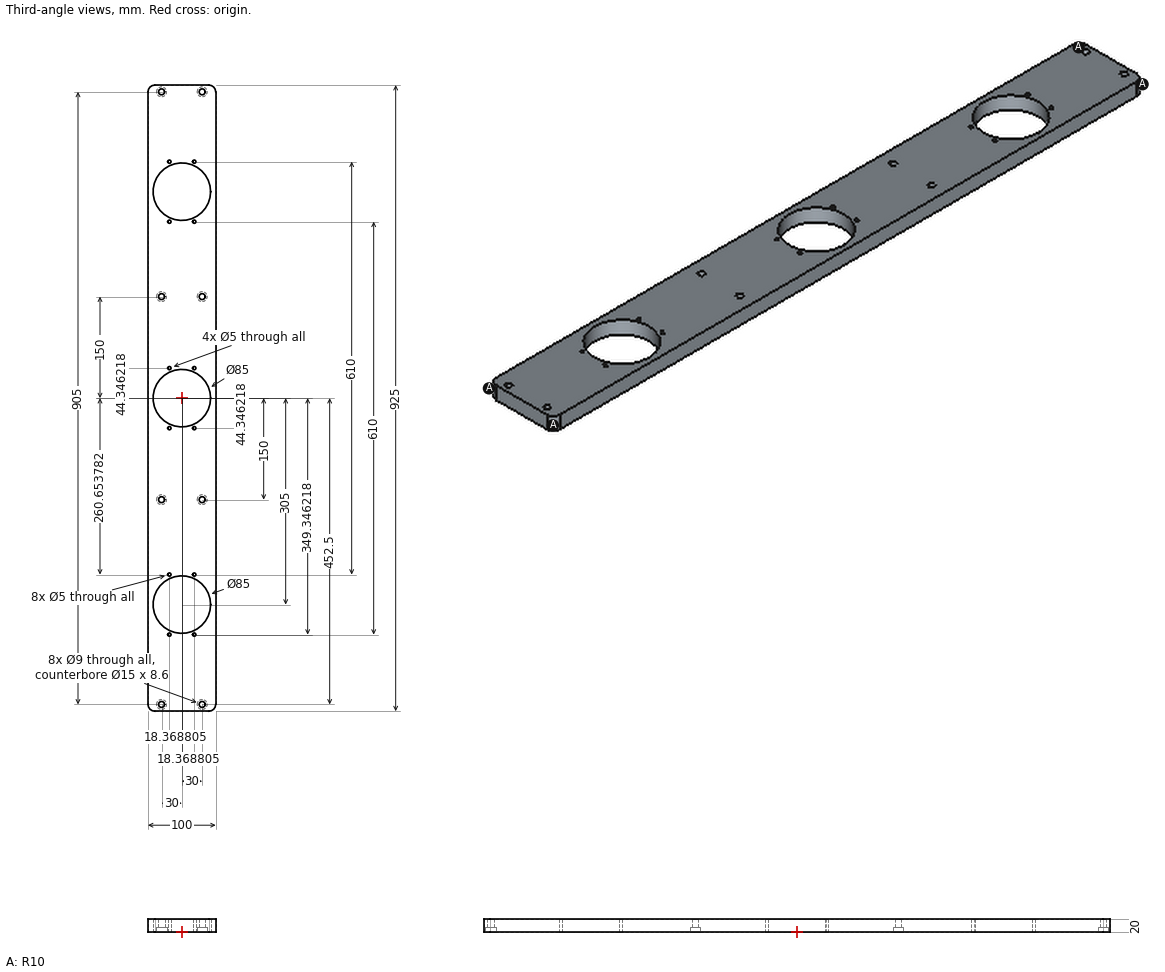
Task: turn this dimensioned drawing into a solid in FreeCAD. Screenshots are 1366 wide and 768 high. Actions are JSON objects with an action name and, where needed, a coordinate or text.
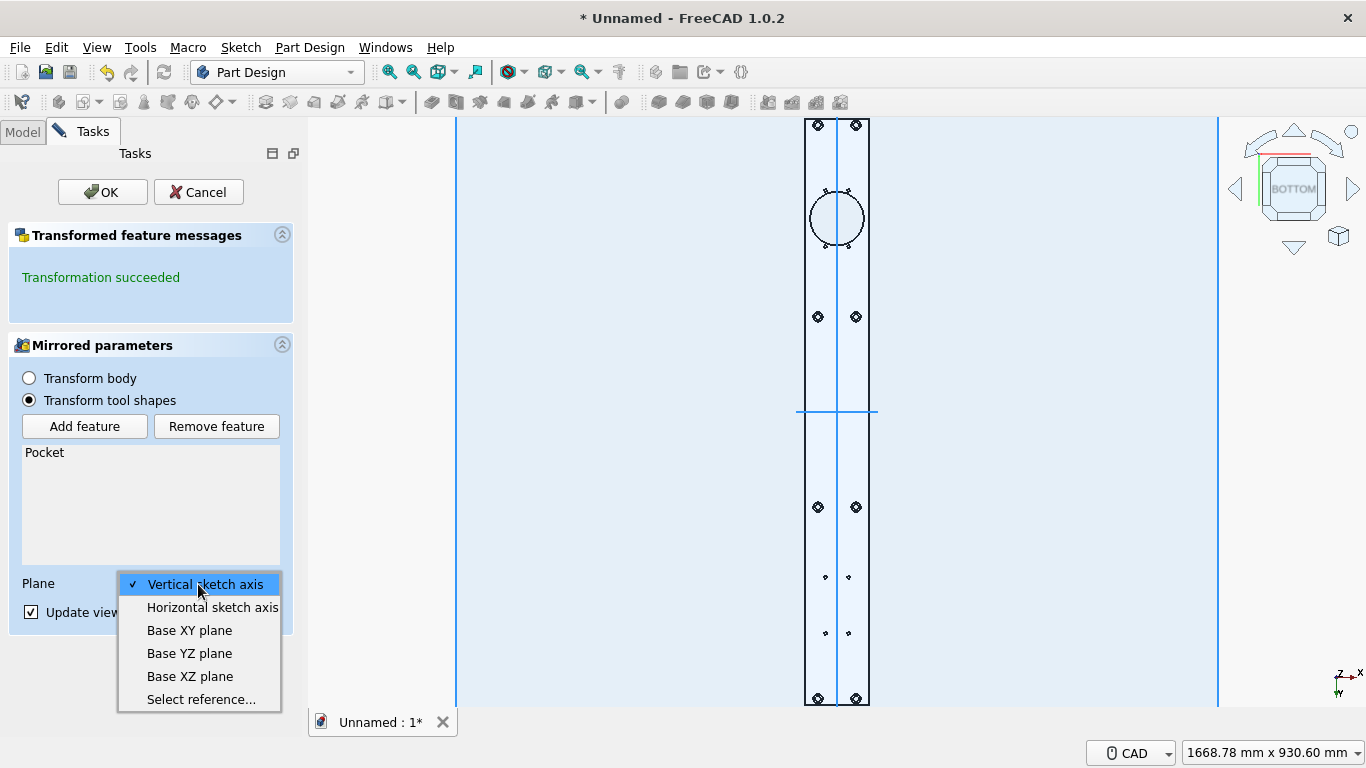
{"action": "left_click", "coordinate": [198, 676]}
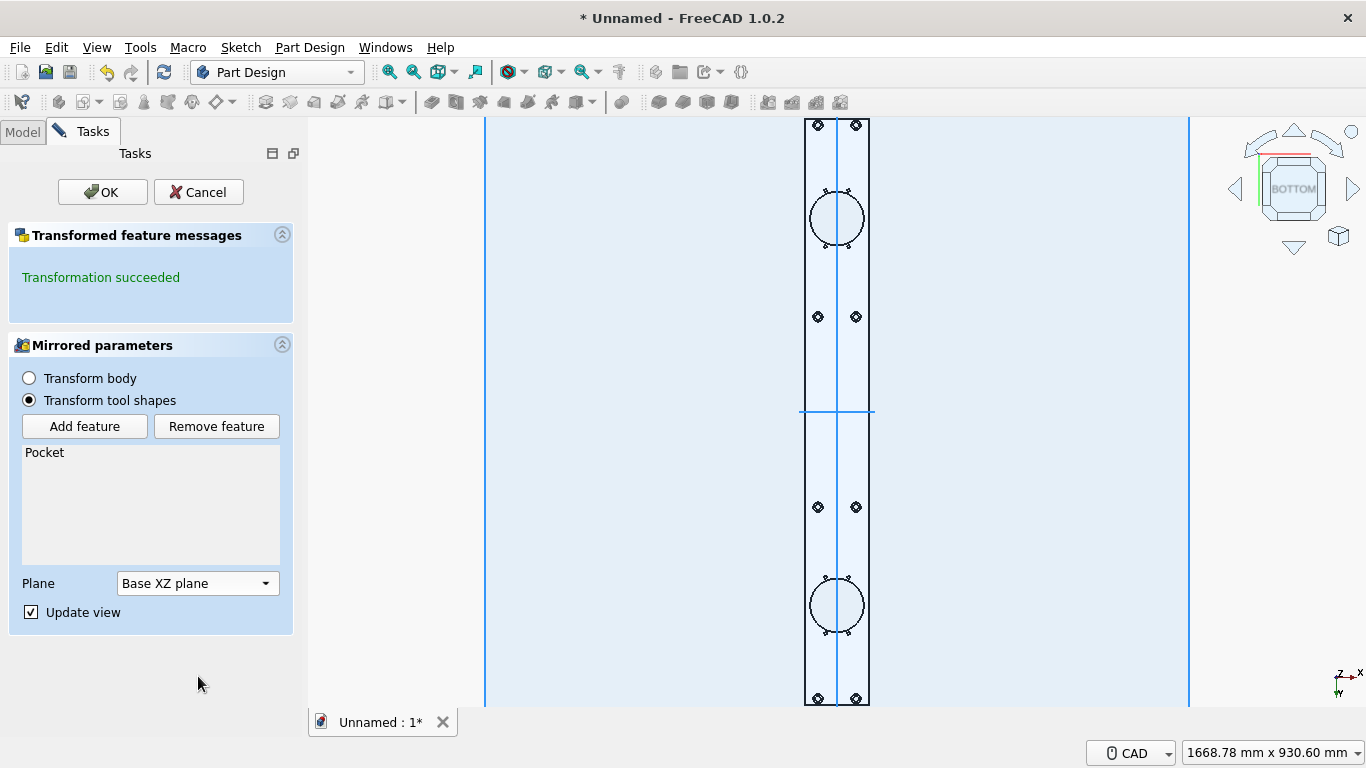
{"action": "left_click", "coordinate": [103, 192]}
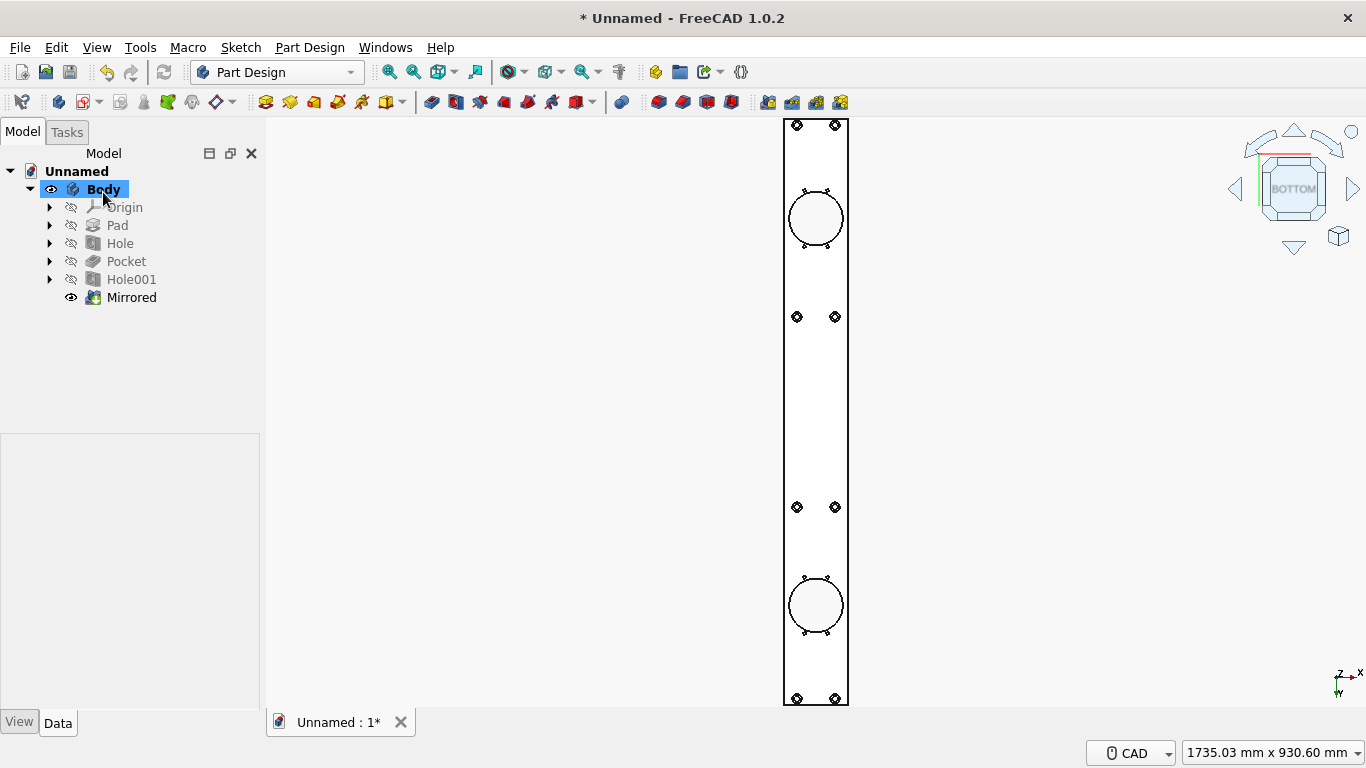
{"action": "key", "text": "0"}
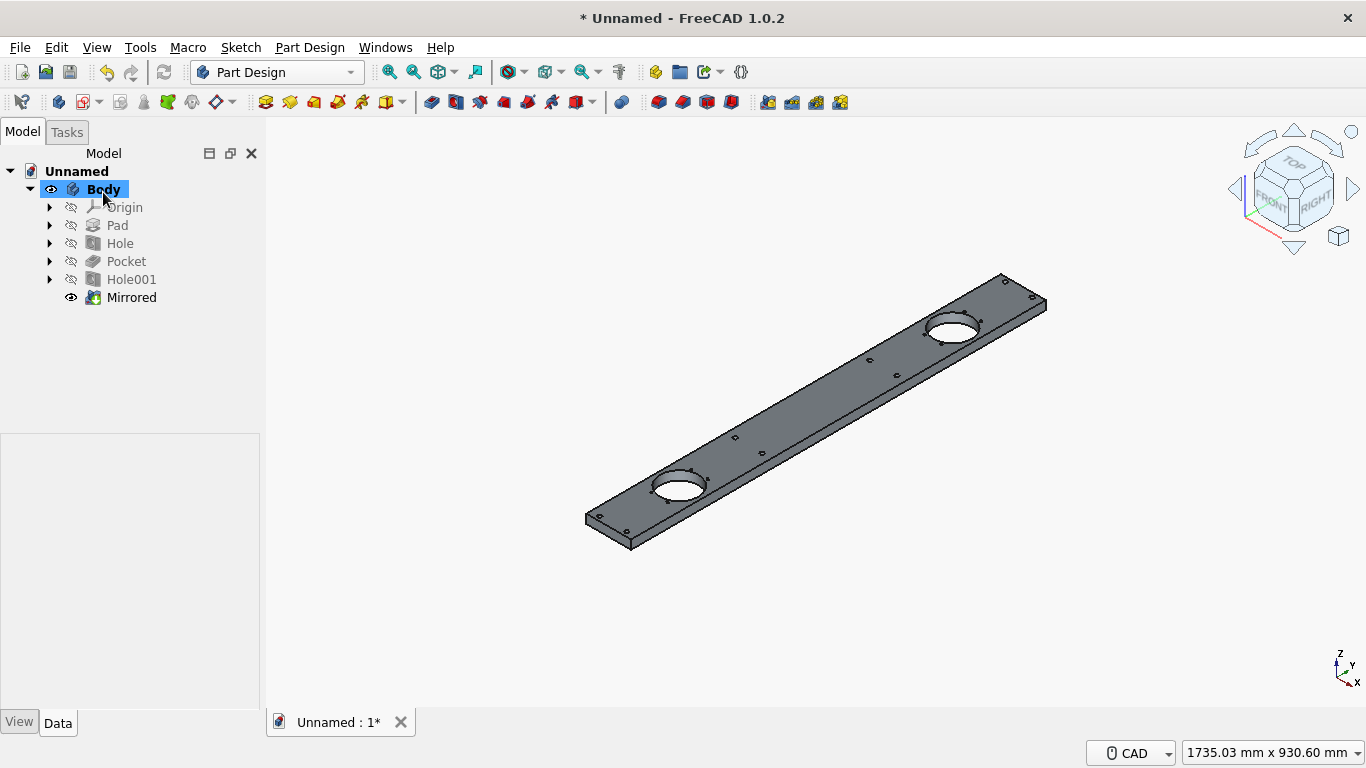
{"action": "left_click", "coordinate": [631, 545]}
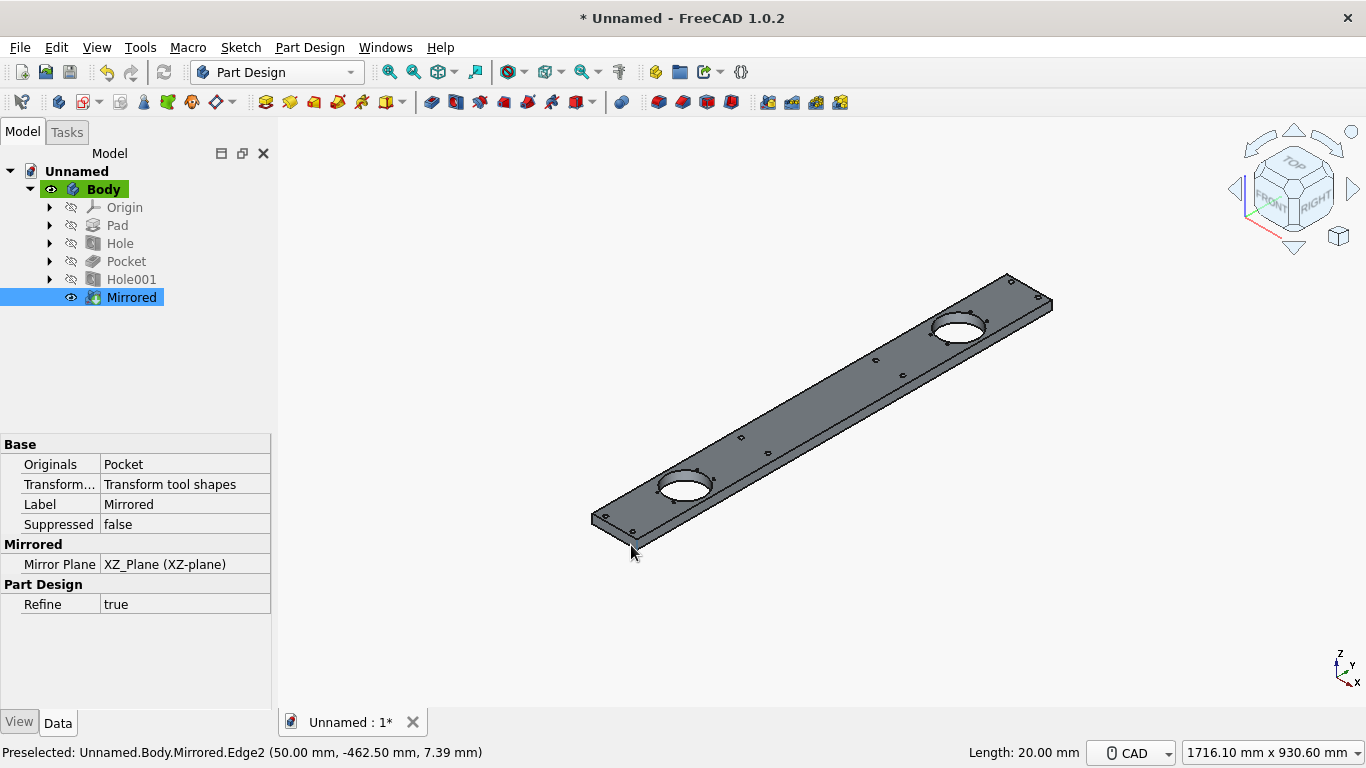
{"action": "scroll", "coordinate": [592, 518], "scroll_direction": "up", "scroll_amount": 6}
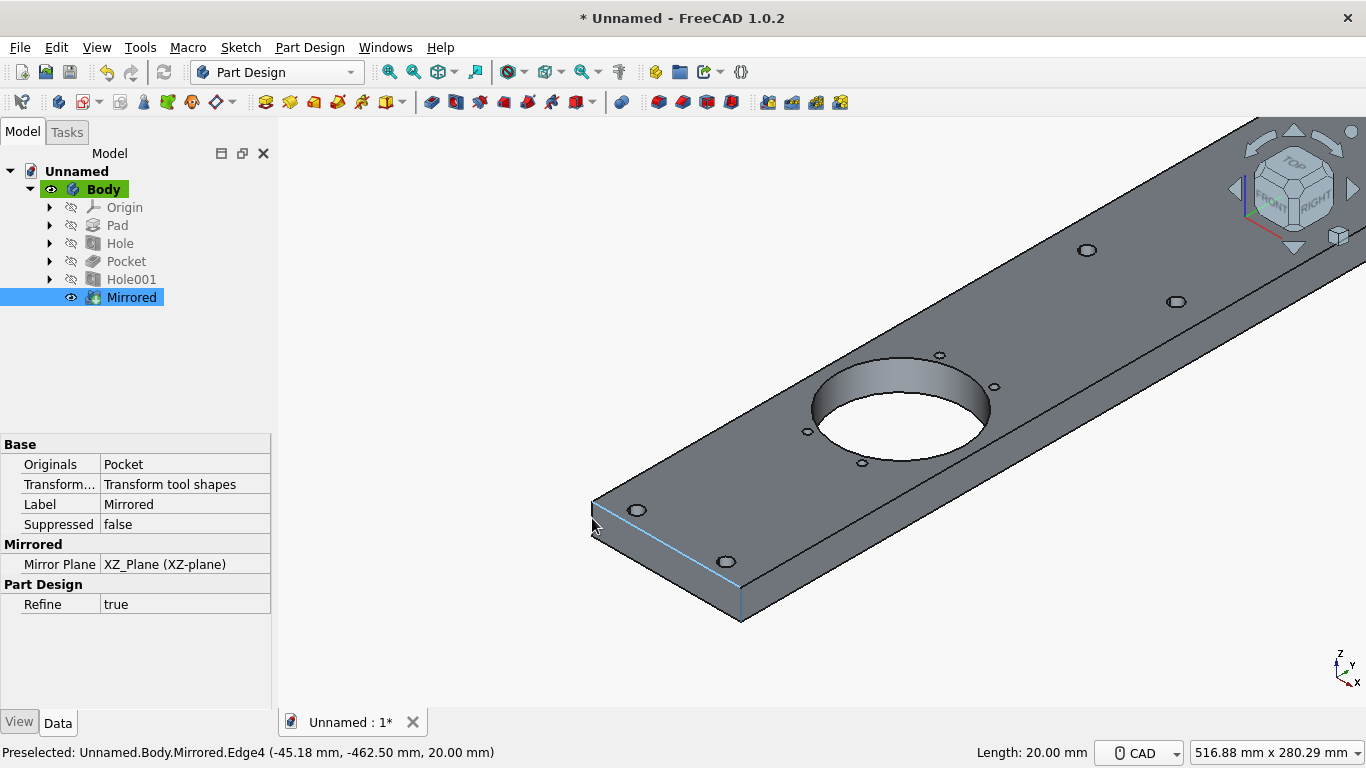
{"action": "left_click", "coordinate": [390, 72]}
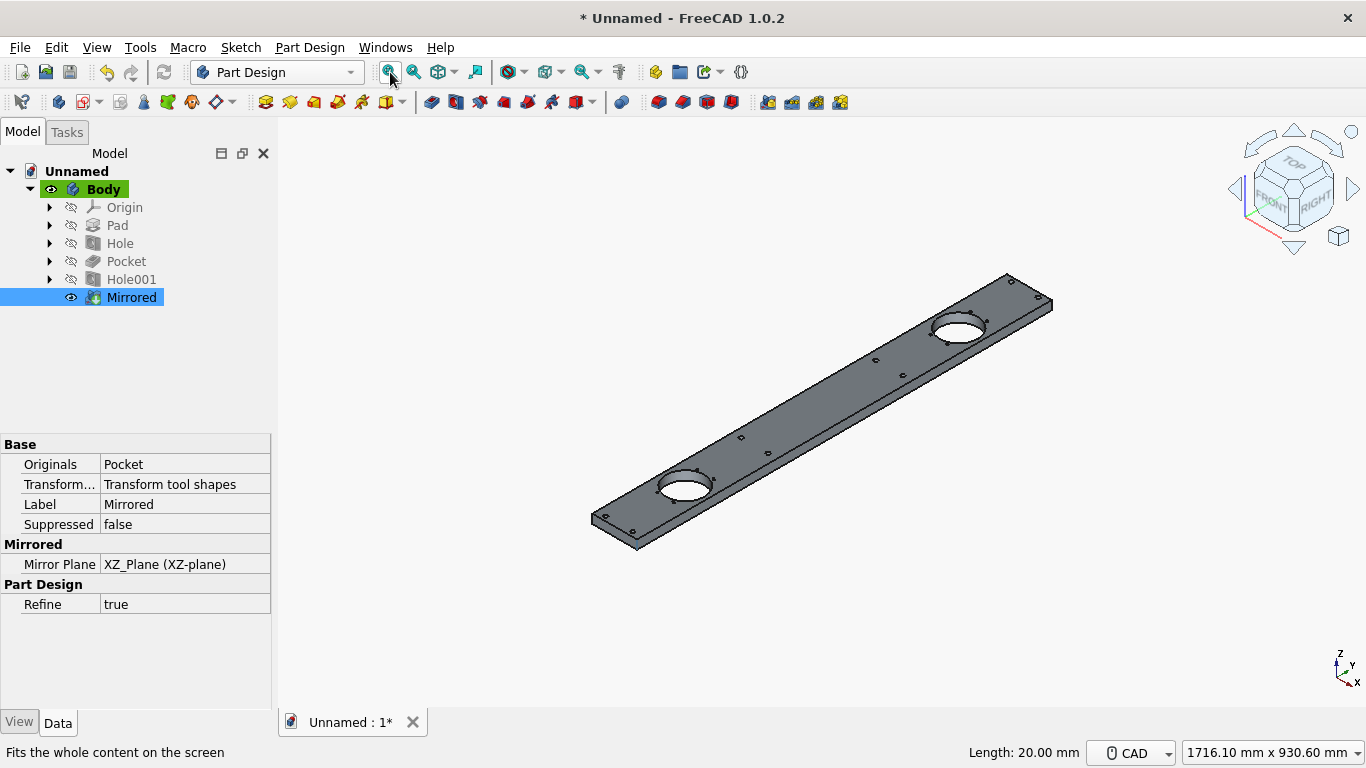
{"action": "key", "text": "2"}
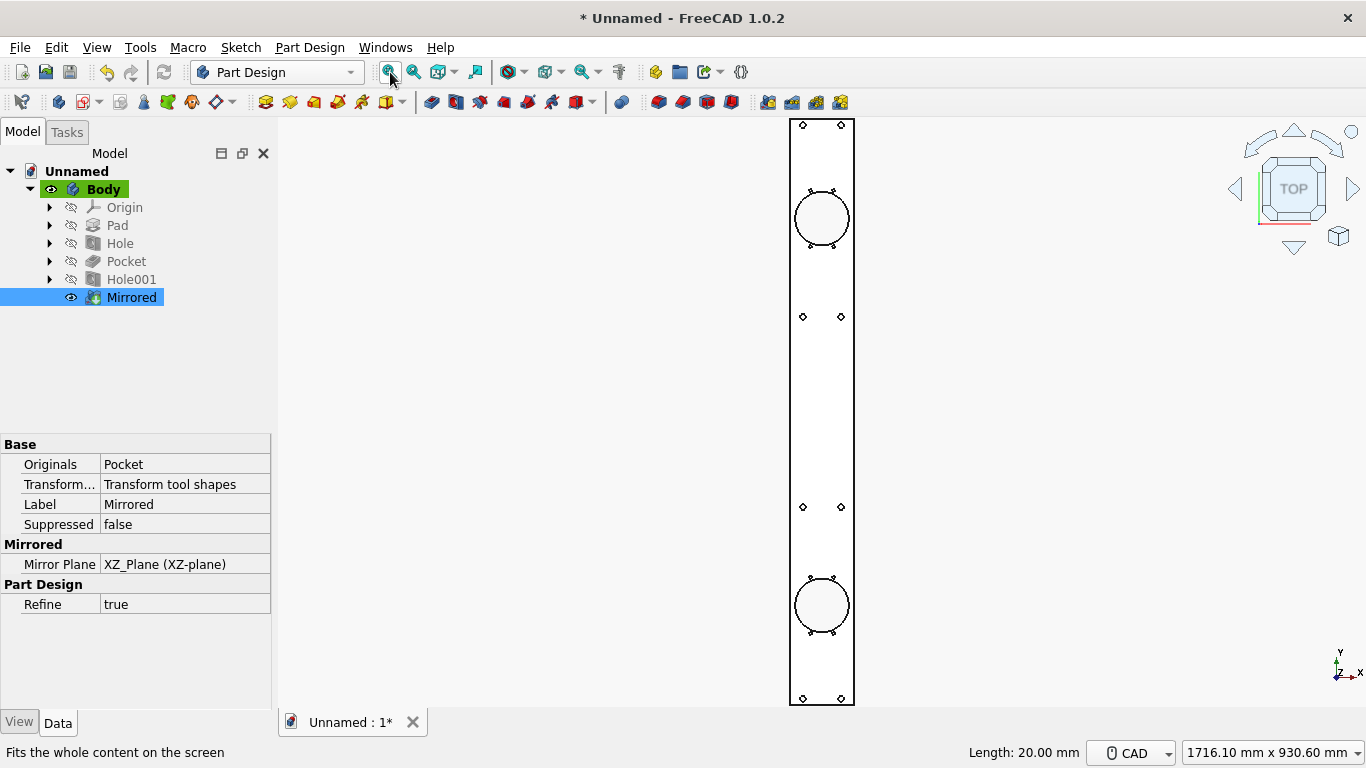
{"action": "key", "text": "1"}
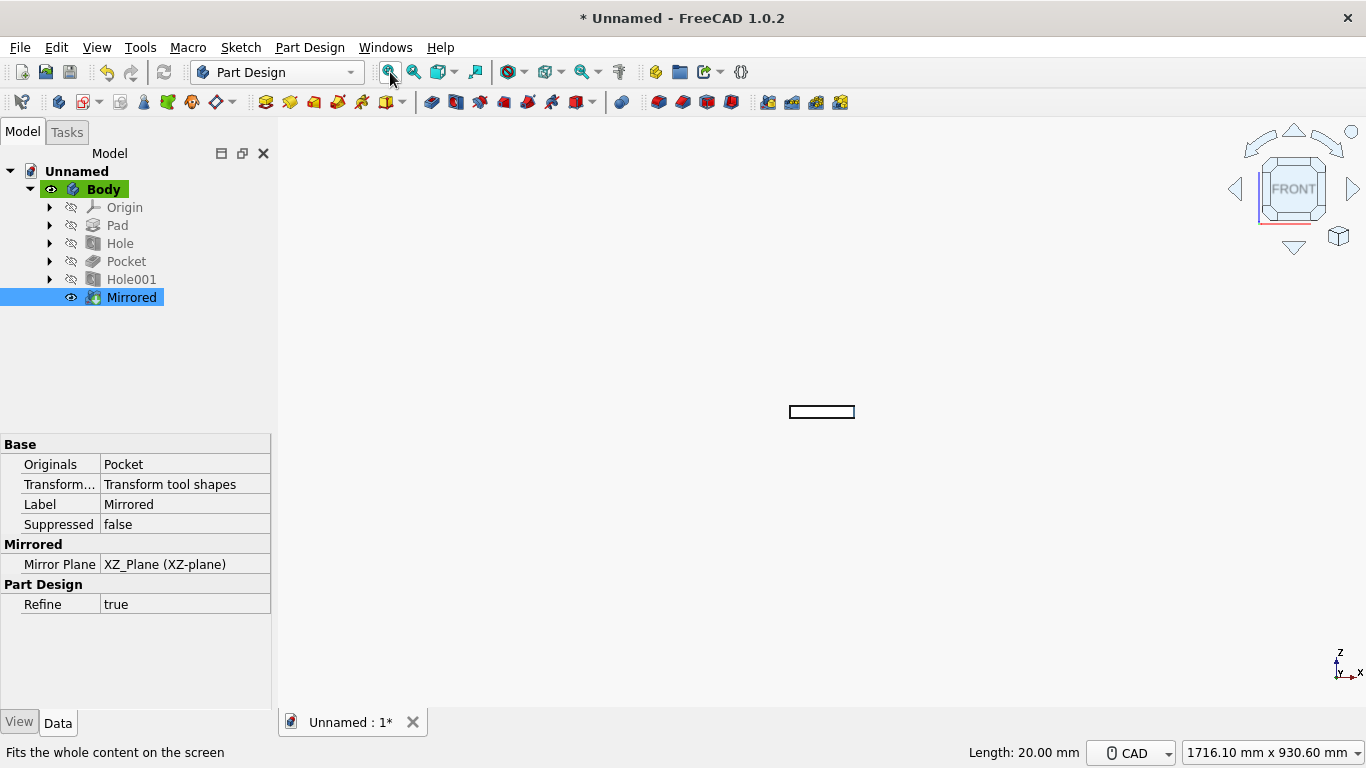
{"action": "key", "text": "v f"}